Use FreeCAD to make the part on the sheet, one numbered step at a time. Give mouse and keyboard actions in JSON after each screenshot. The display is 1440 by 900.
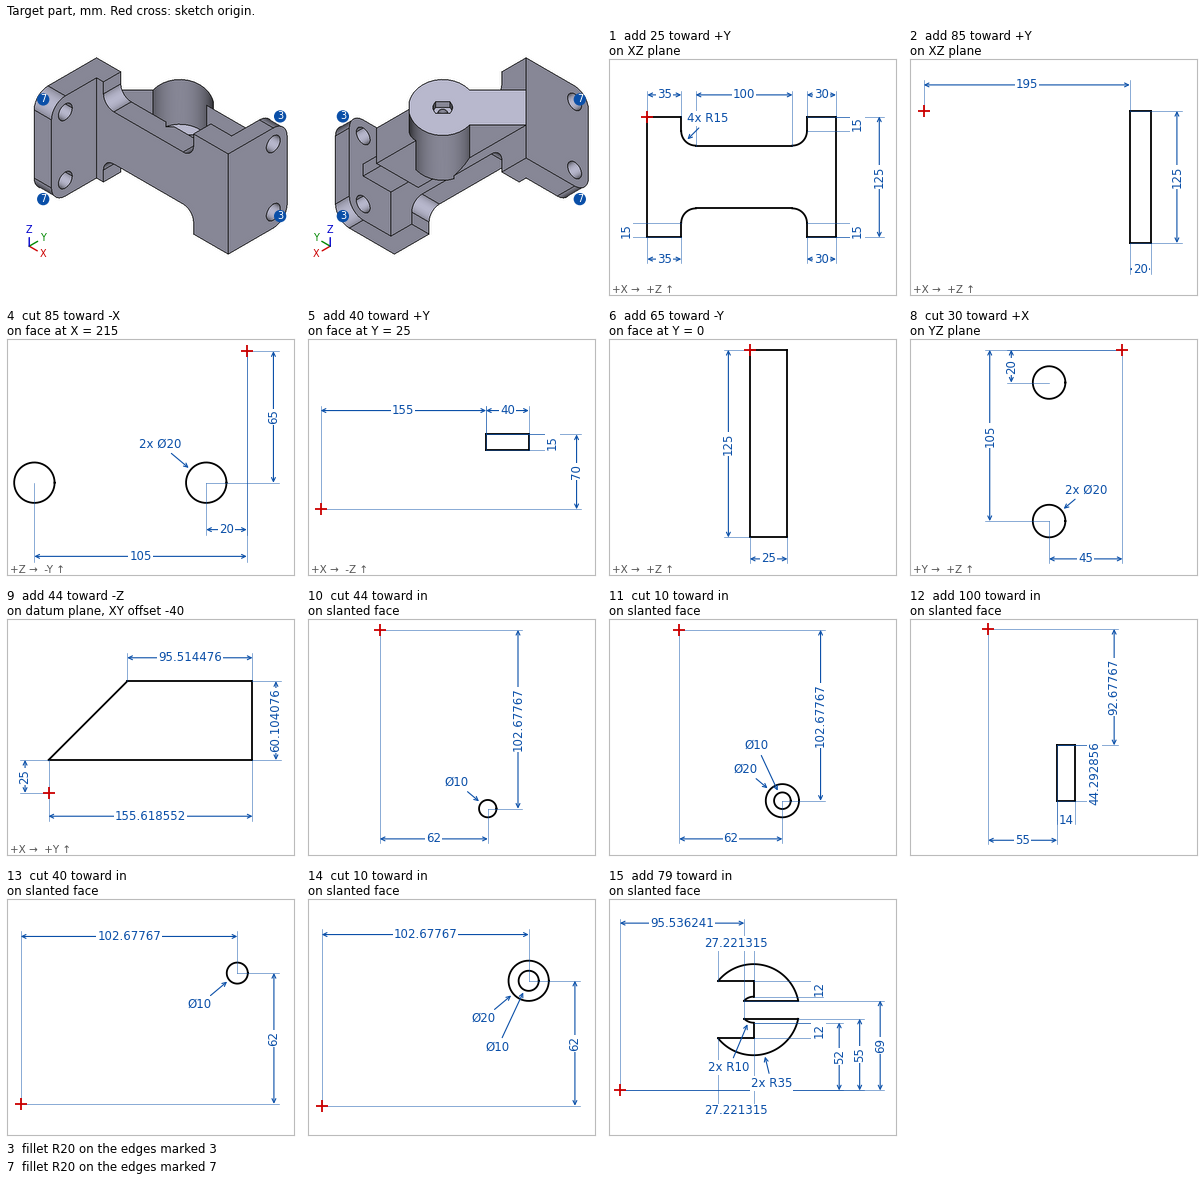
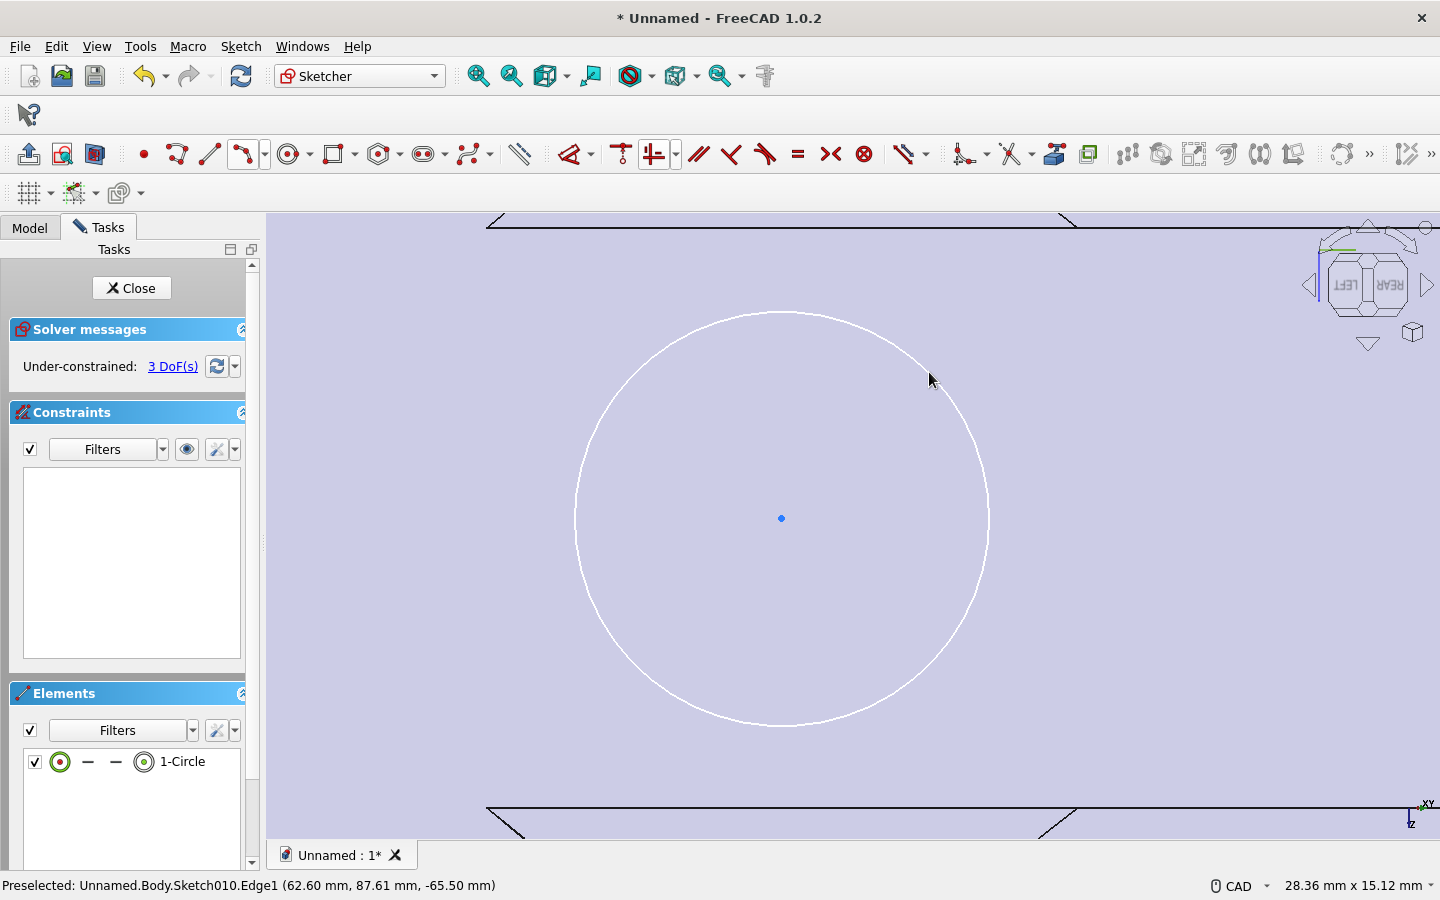
{"action": "left_click", "coordinate": [568, 154]}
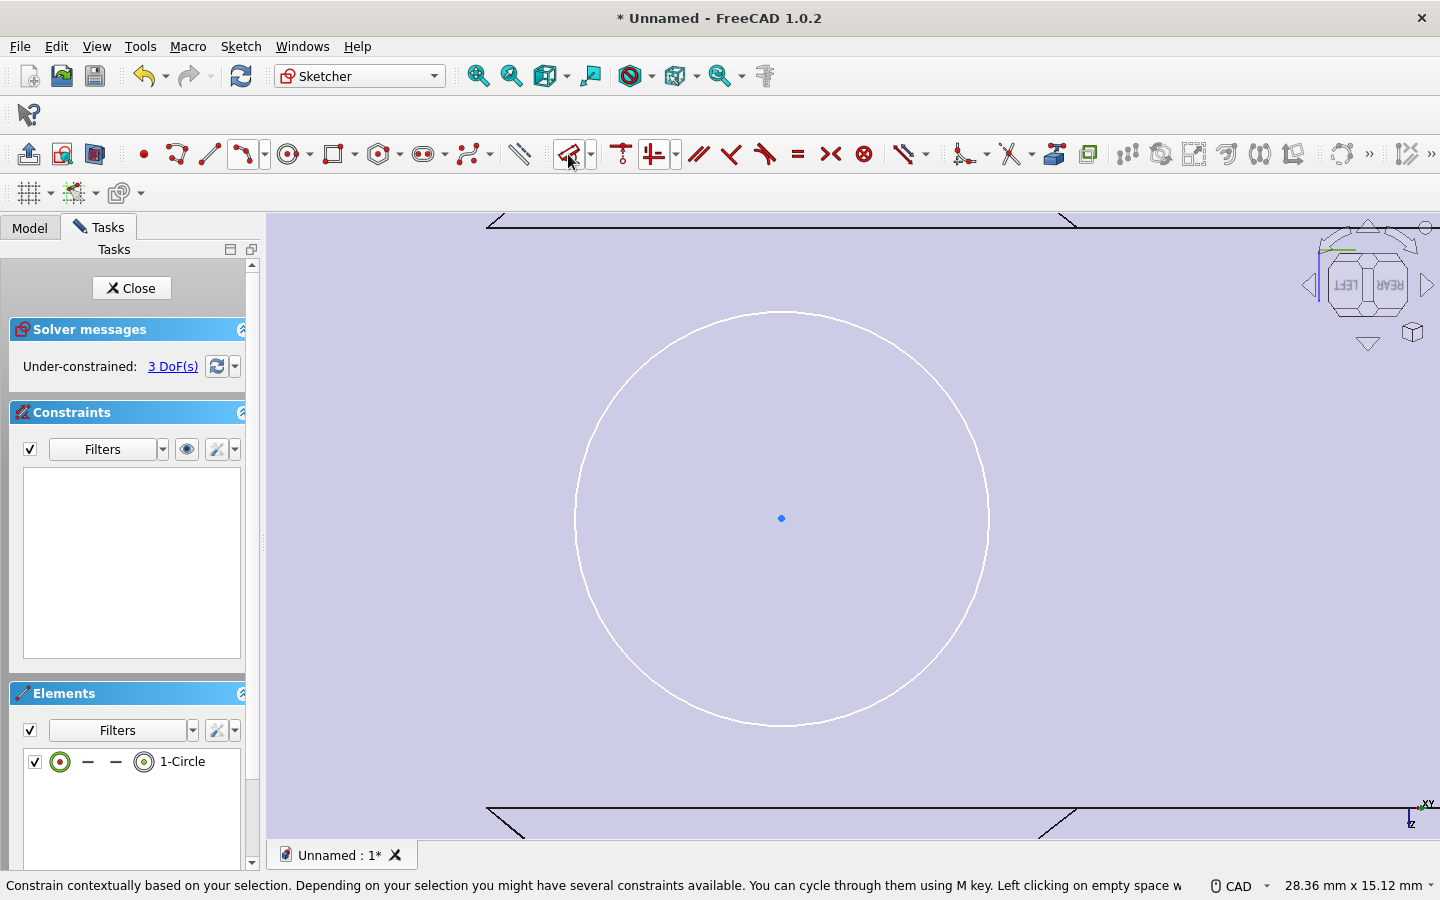
{"action": "left_click", "coordinate": [928, 372]}
{"action": "left_click", "coordinate": [951, 349]}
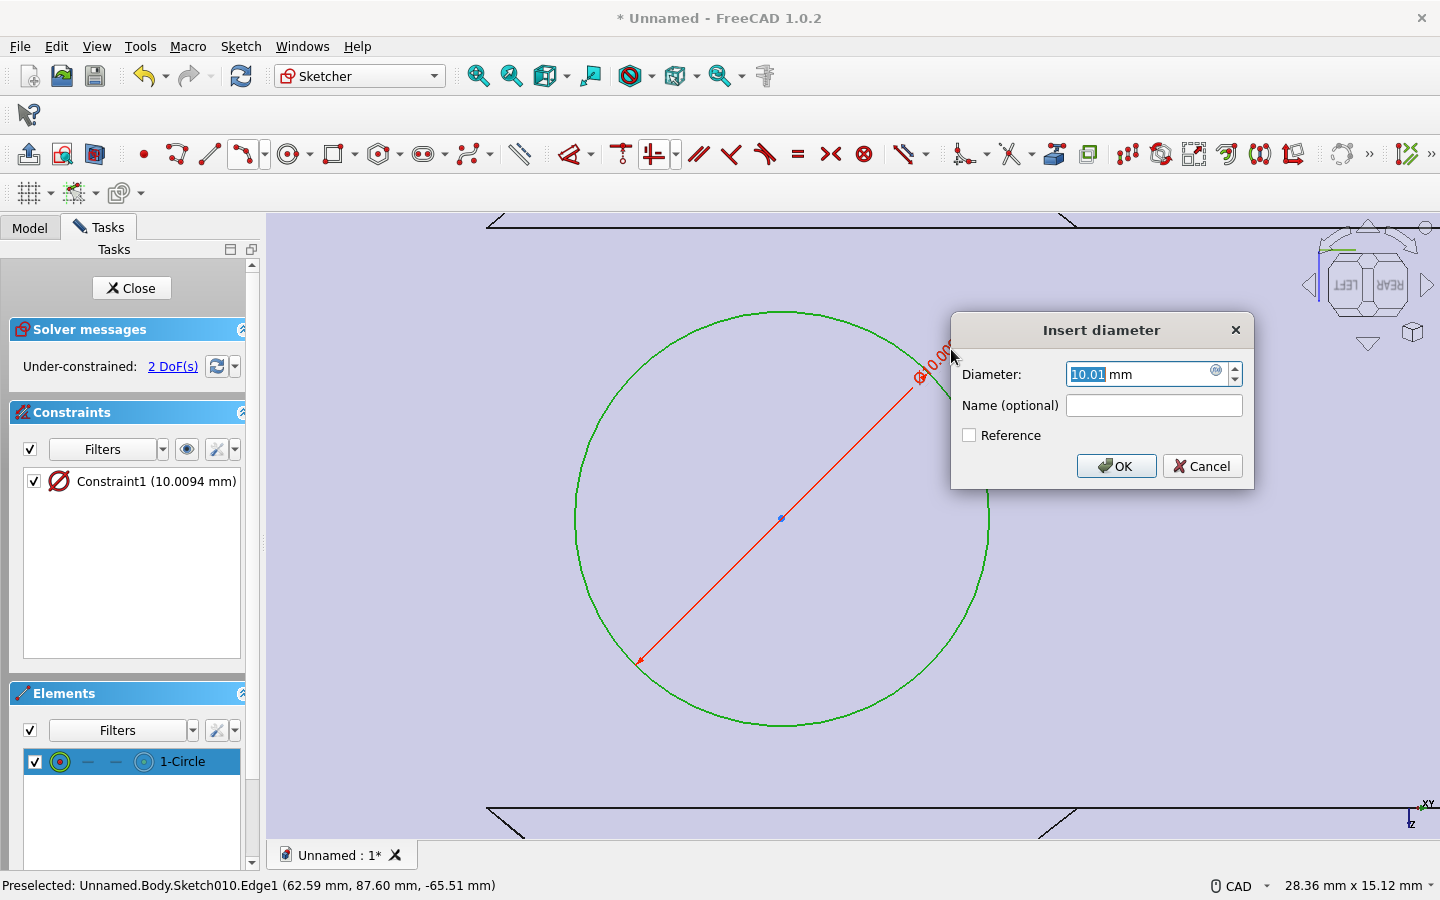
{"action": "type", "text": "10"}
{"action": "key", "text": "Return"}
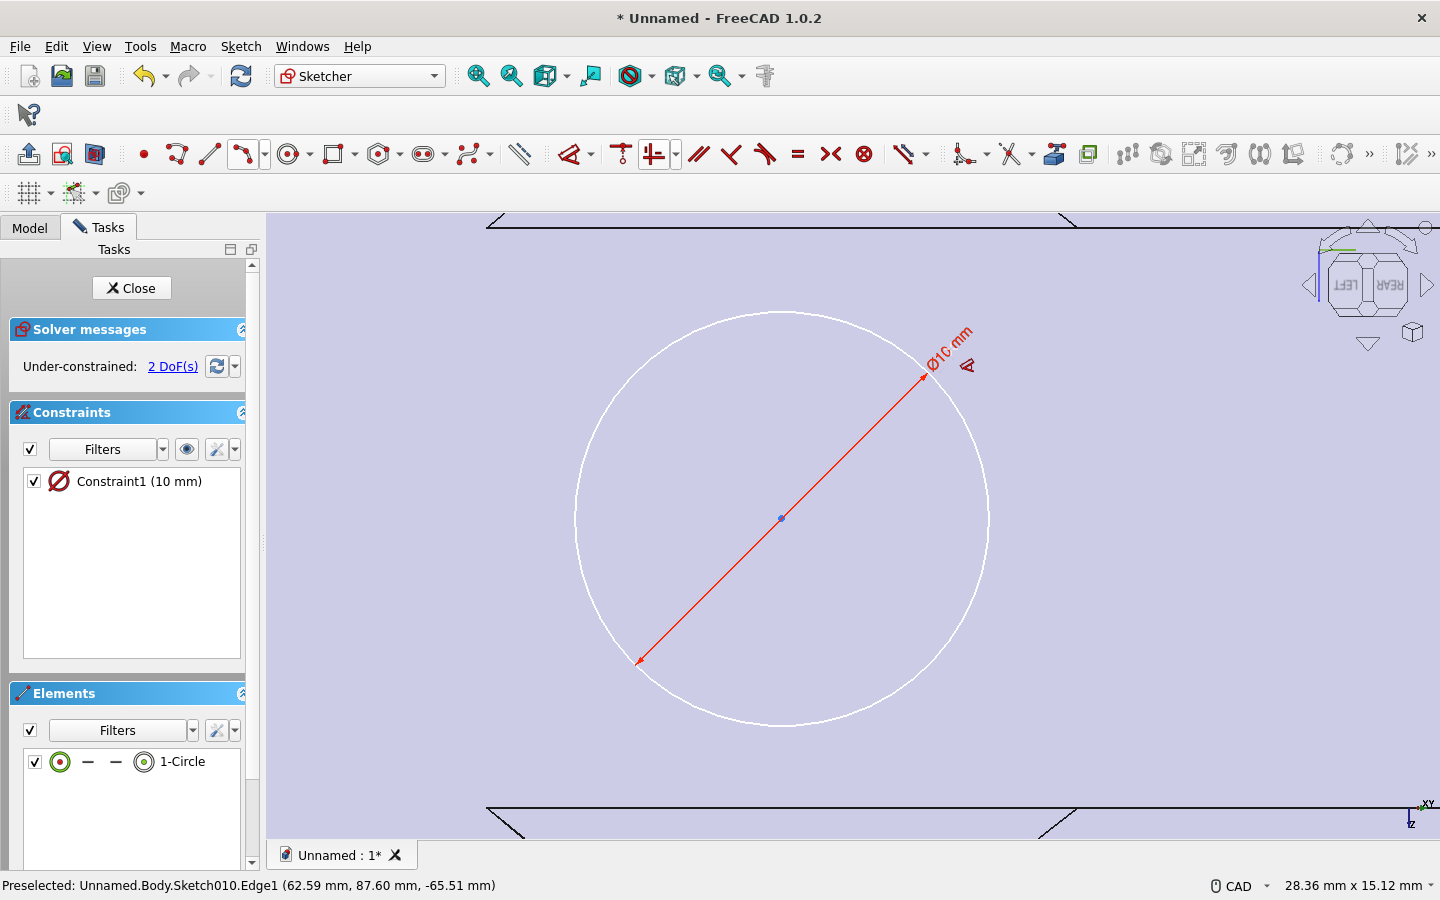
{"action": "left_click", "coordinate": [782, 519]}
{"action": "left_click", "coordinate": [816, 665]}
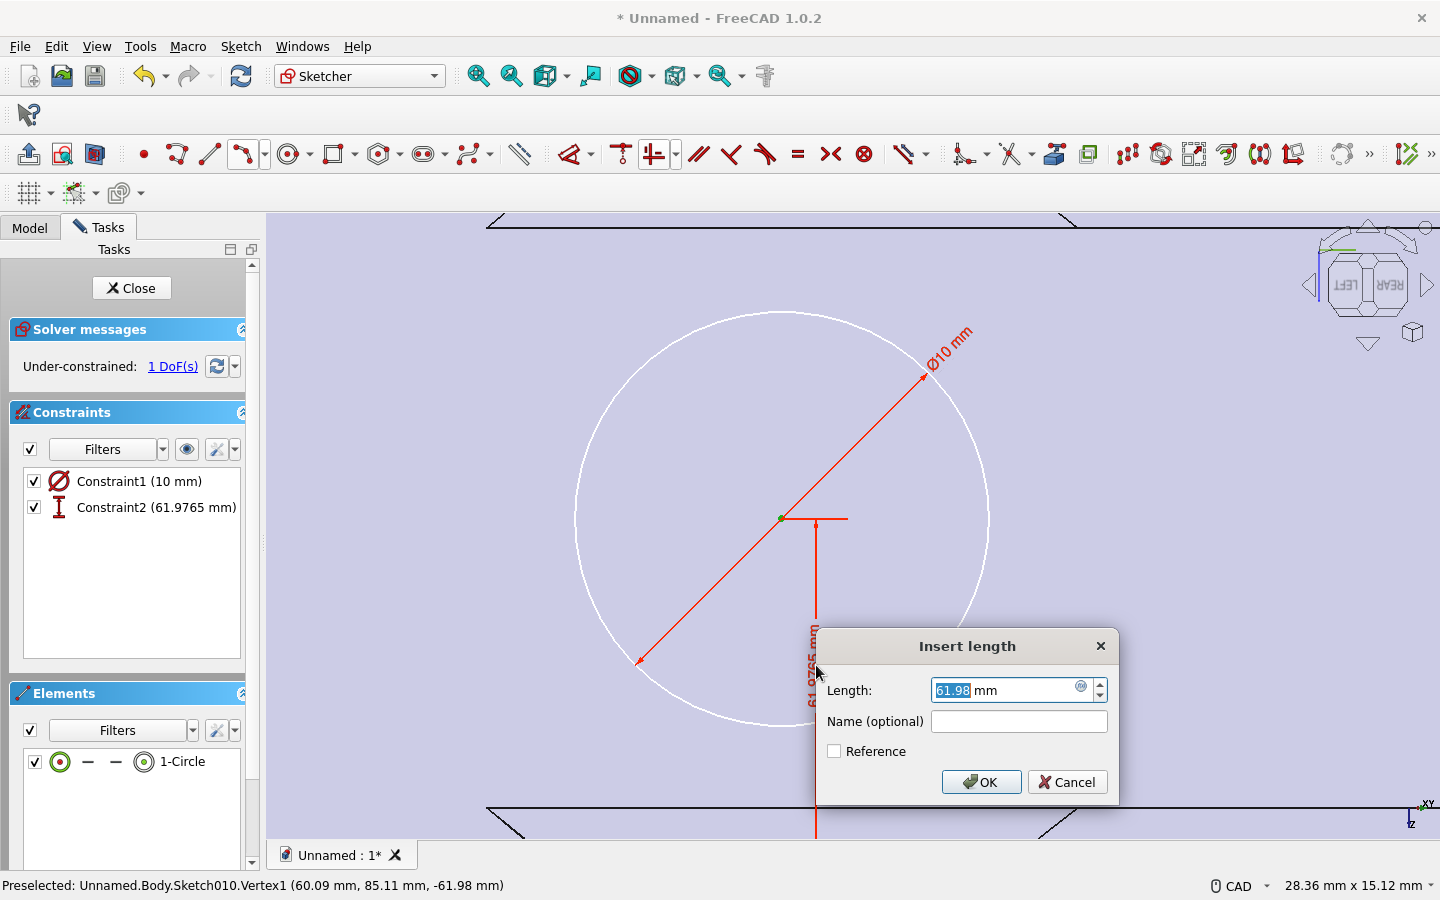
{"action": "type", "text": "62"}
{"action": "key", "text": "Return"}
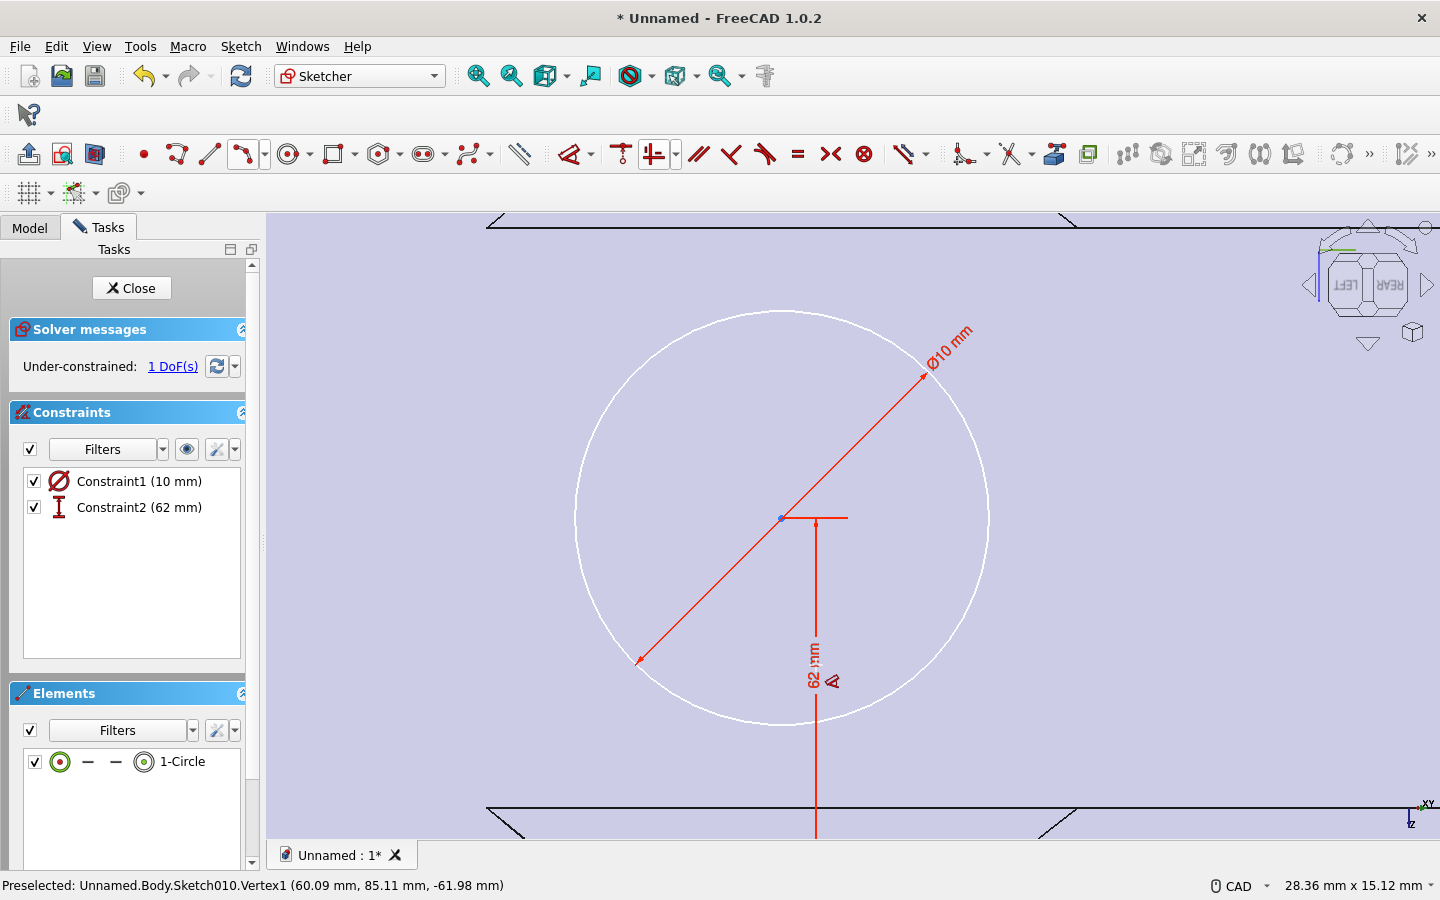
{"action": "left_click", "coordinate": [782, 518]}
{"action": "left_click", "coordinate": [538, 484]}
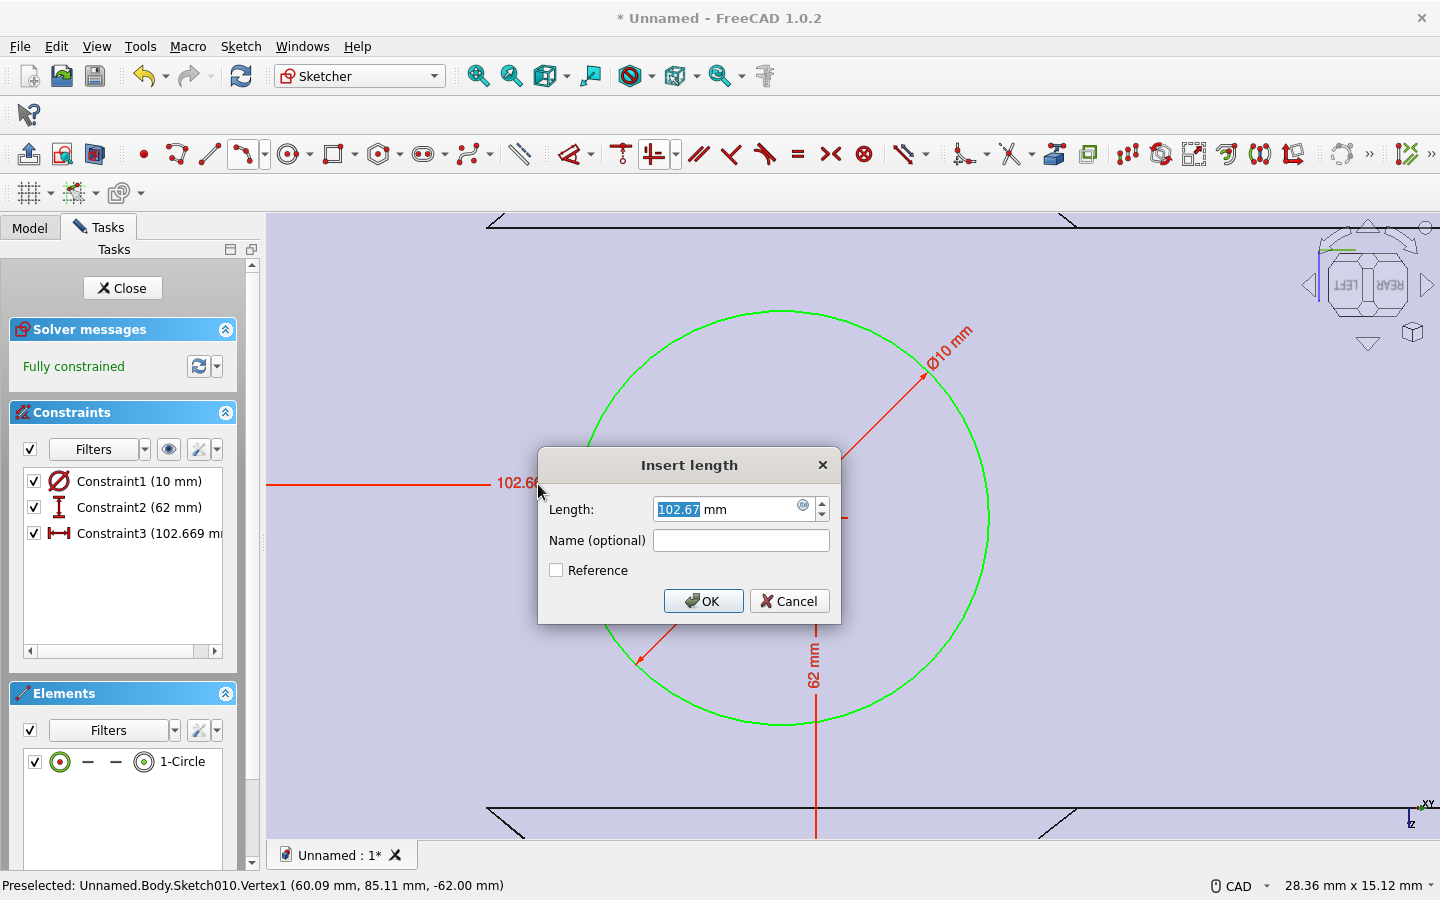
{"action": "type", "text": "102.67767"}
{"action": "key", "text": "Return"}
{"action": "key", "text": "Escape"}